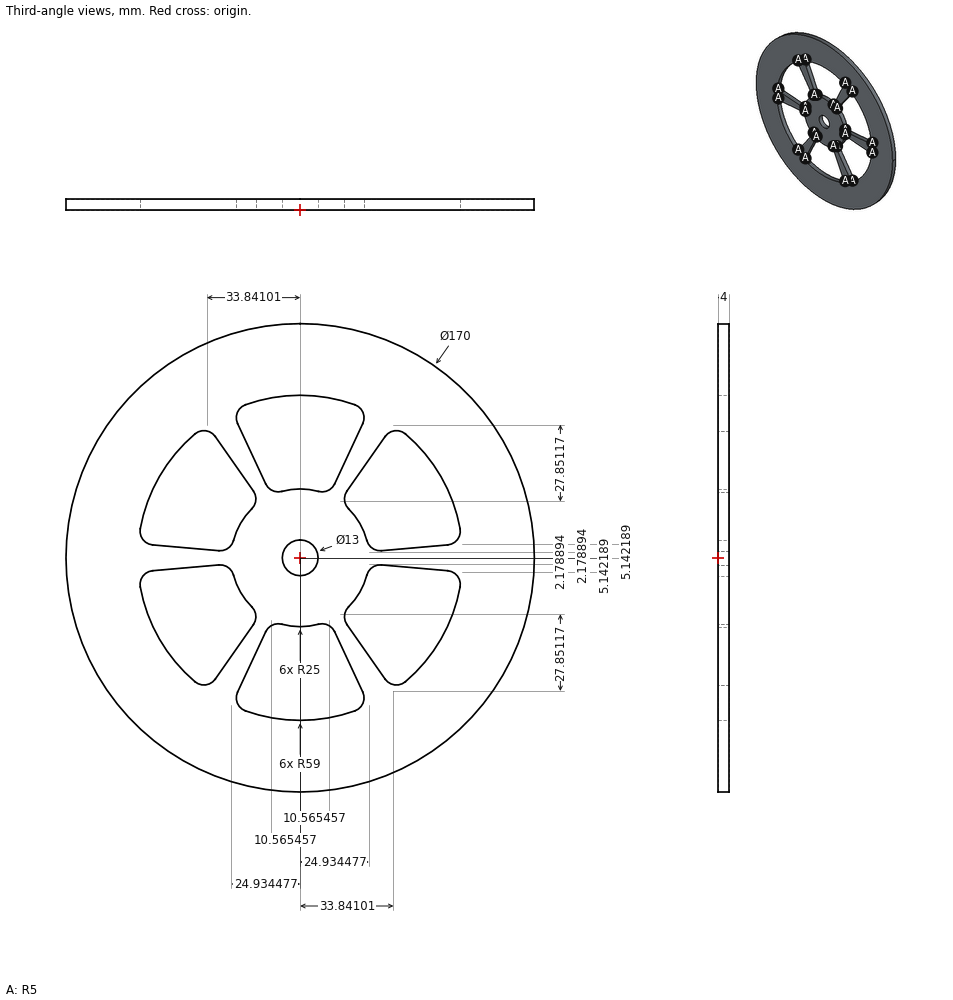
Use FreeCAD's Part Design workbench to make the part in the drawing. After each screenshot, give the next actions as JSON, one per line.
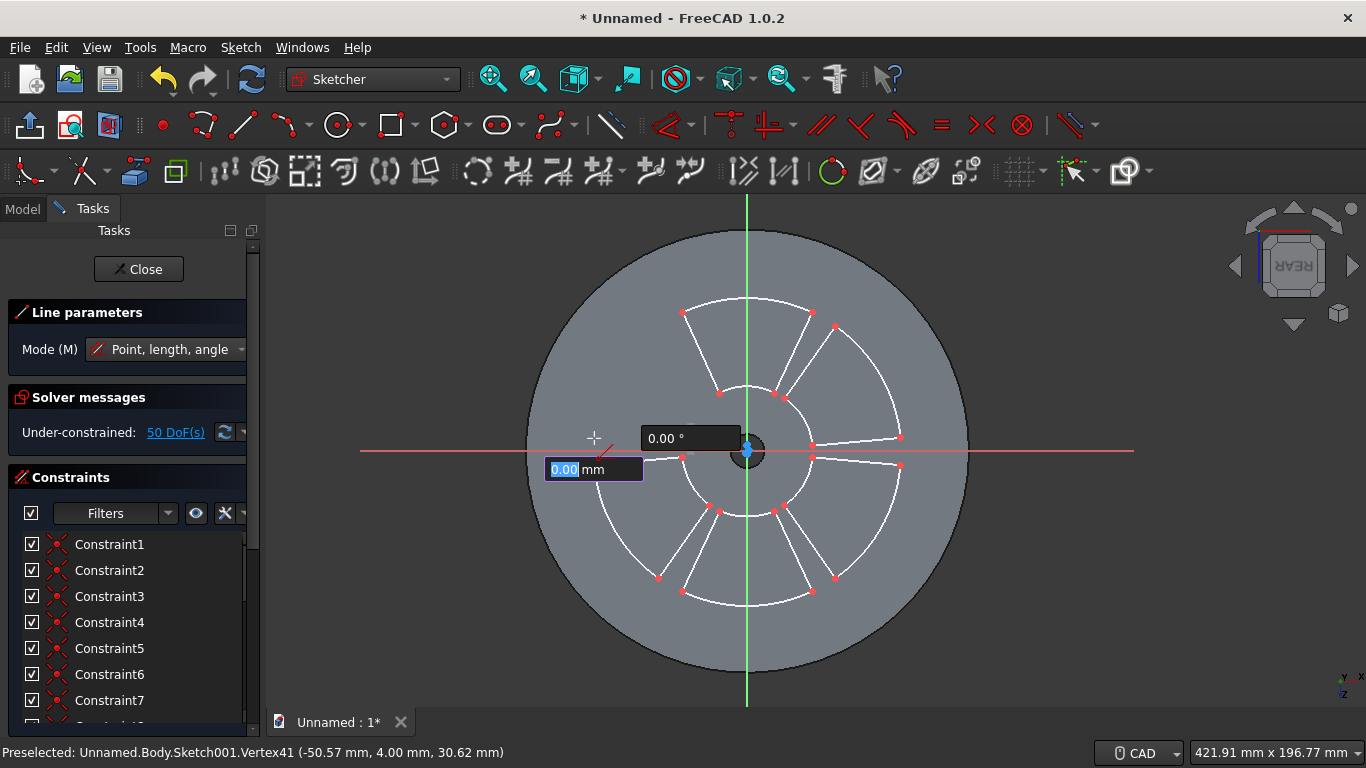
{"action": "scroll", "coordinate": [682, 445], "scroll_direction": "up", "scroll_amount": 6}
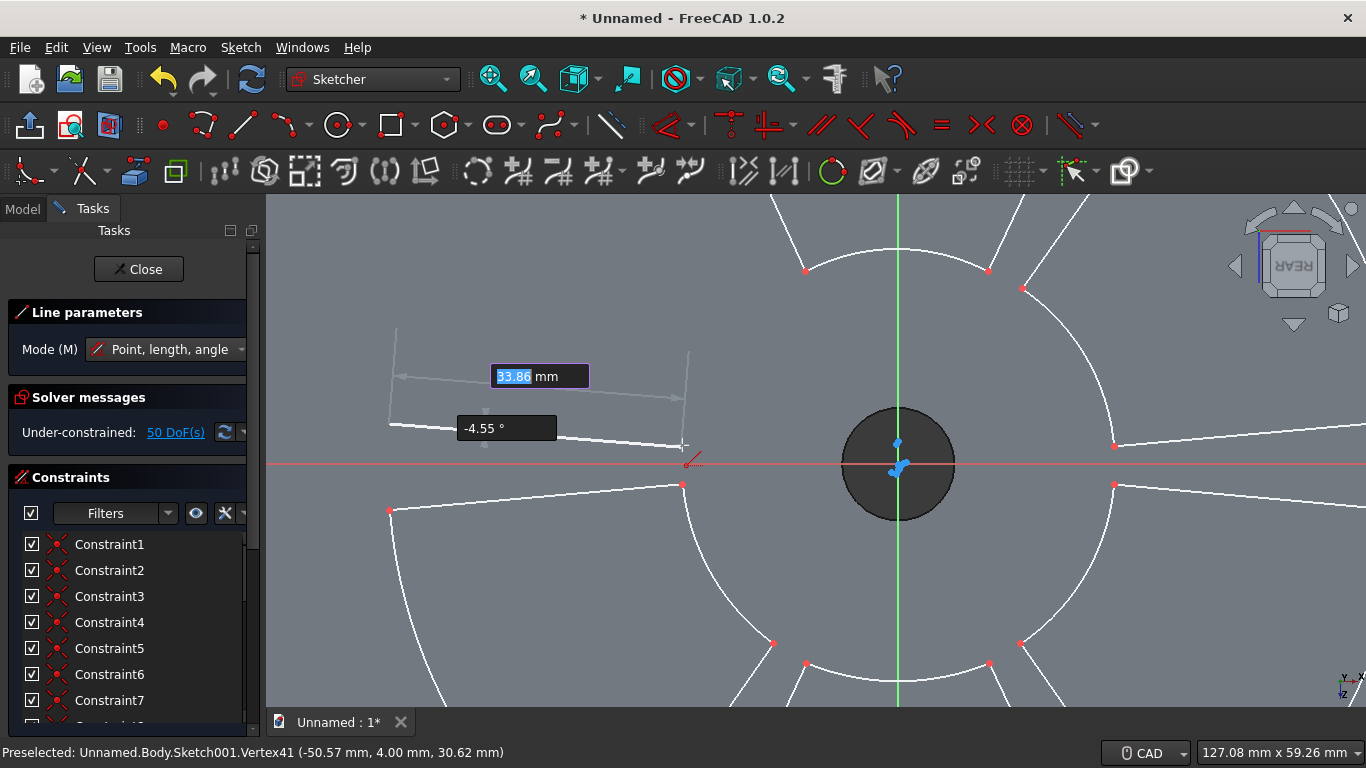
{"action": "left_click", "coordinate": [683, 445]}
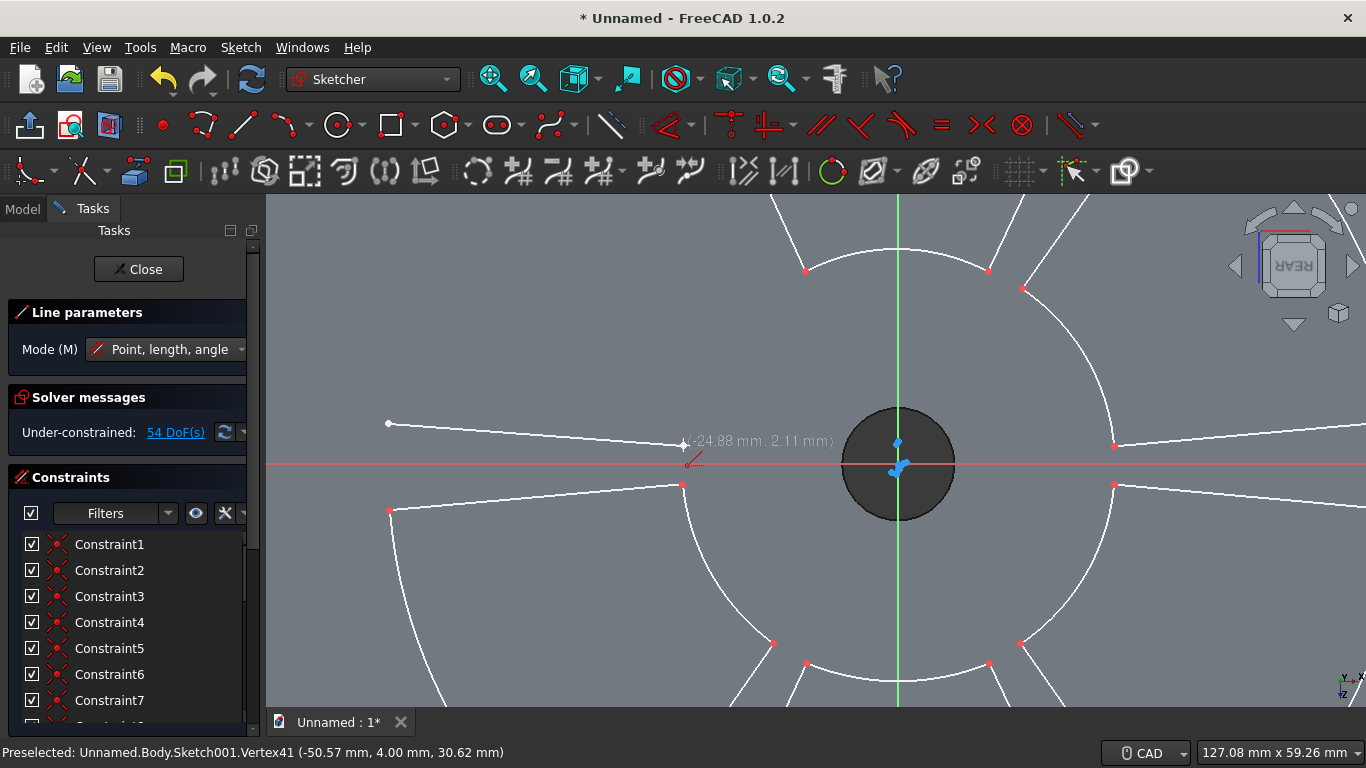
{"action": "left_click", "coordinate": [774, 287]}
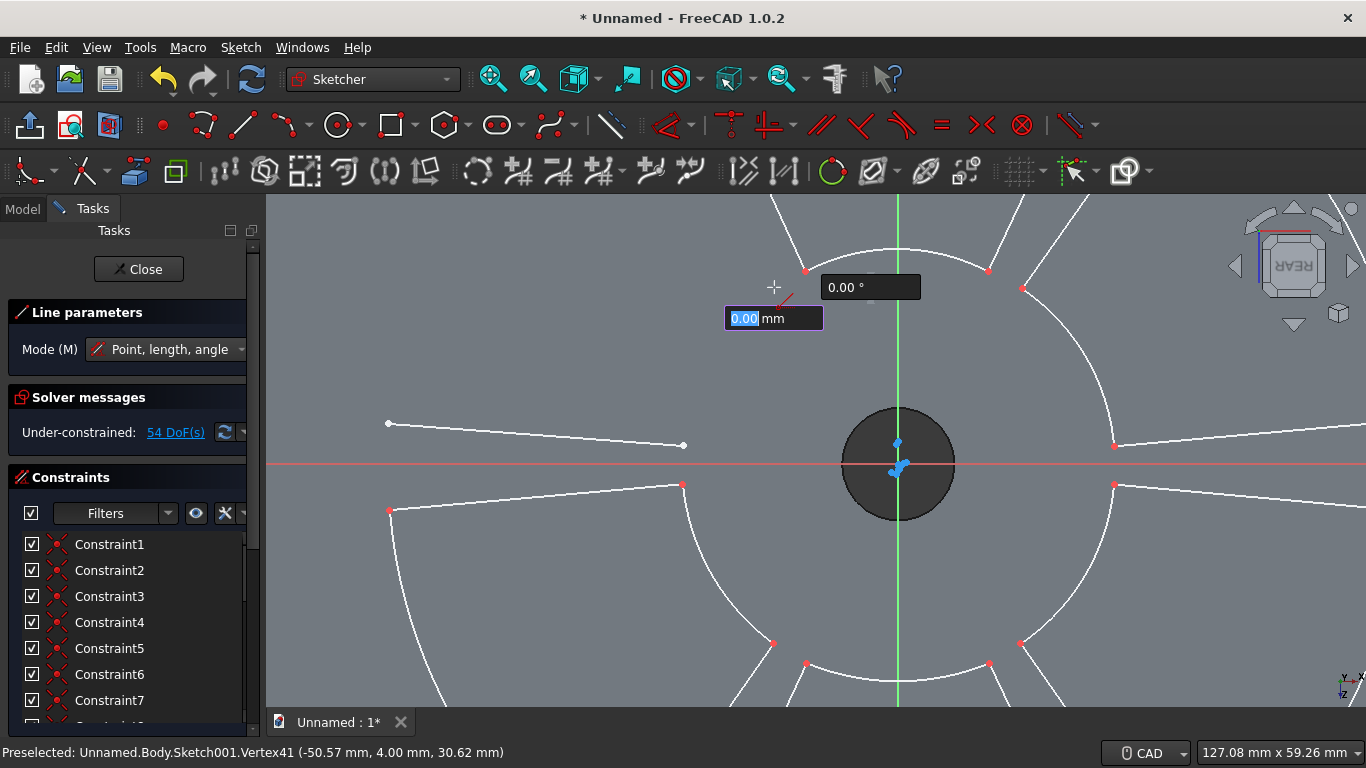
{"action": "scroll", "coordinate": [682, 445], "scroll_direction": "down", "scroll_amount": 6}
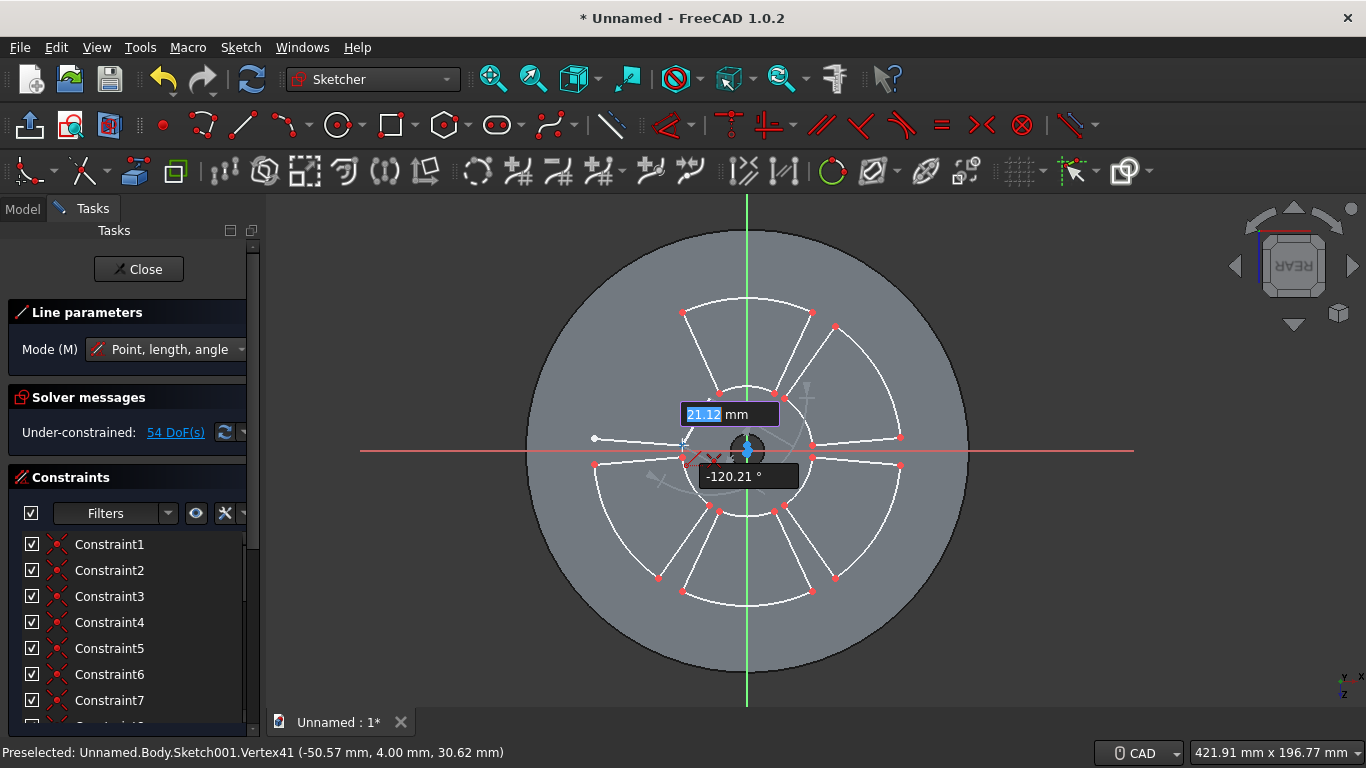
{"action": "left_click", "coordinate": [659, 325]}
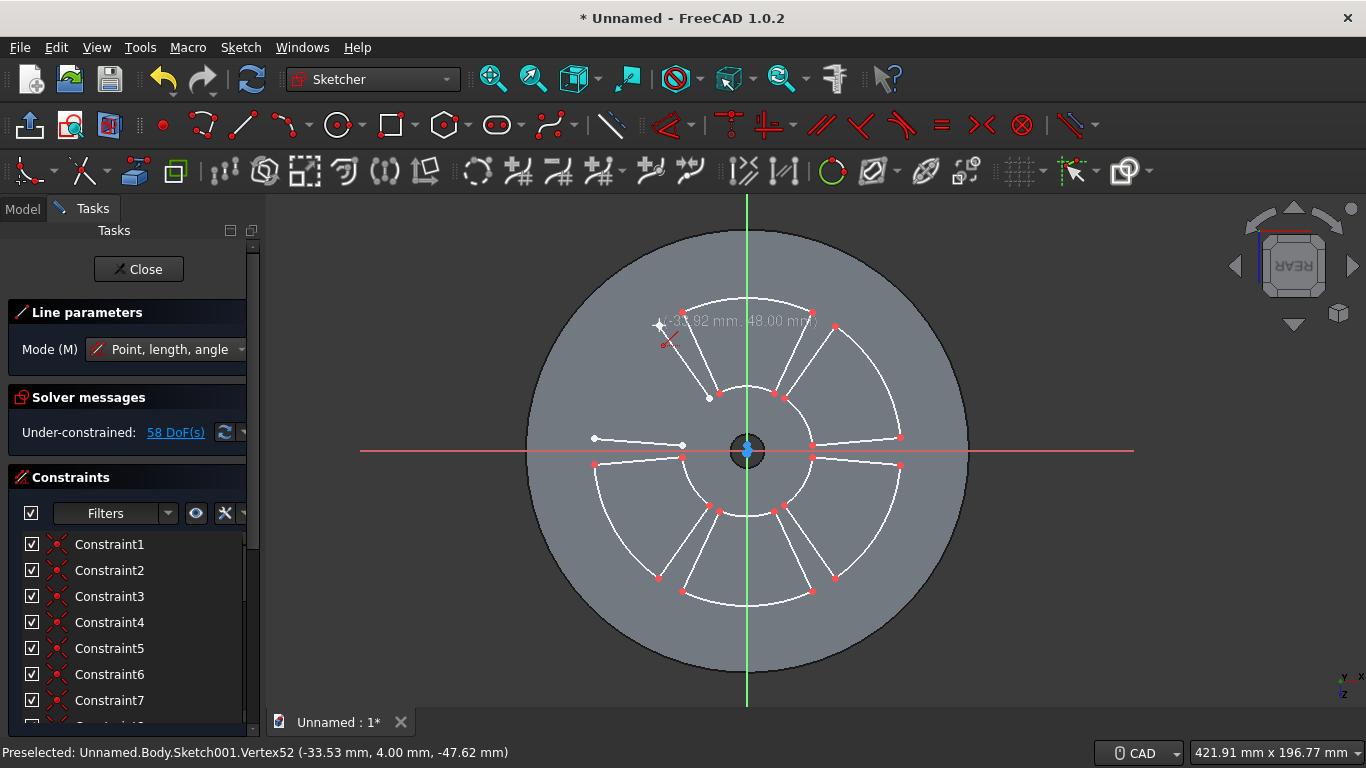
{"action": "left_click", "coordinate": [284, 126]}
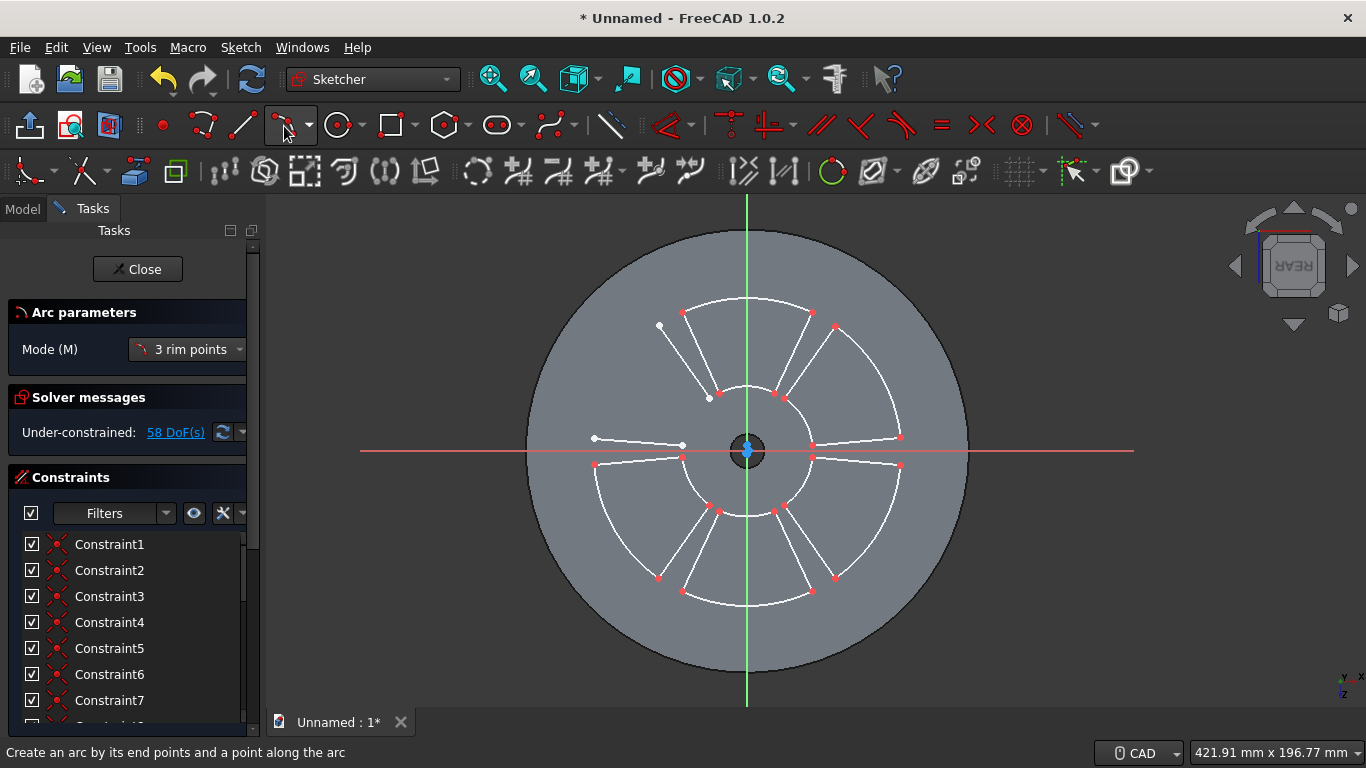
{"action": "scroll", "coordinate": [682, 445], "scroll_direction": "up", "scroll_amount": 6}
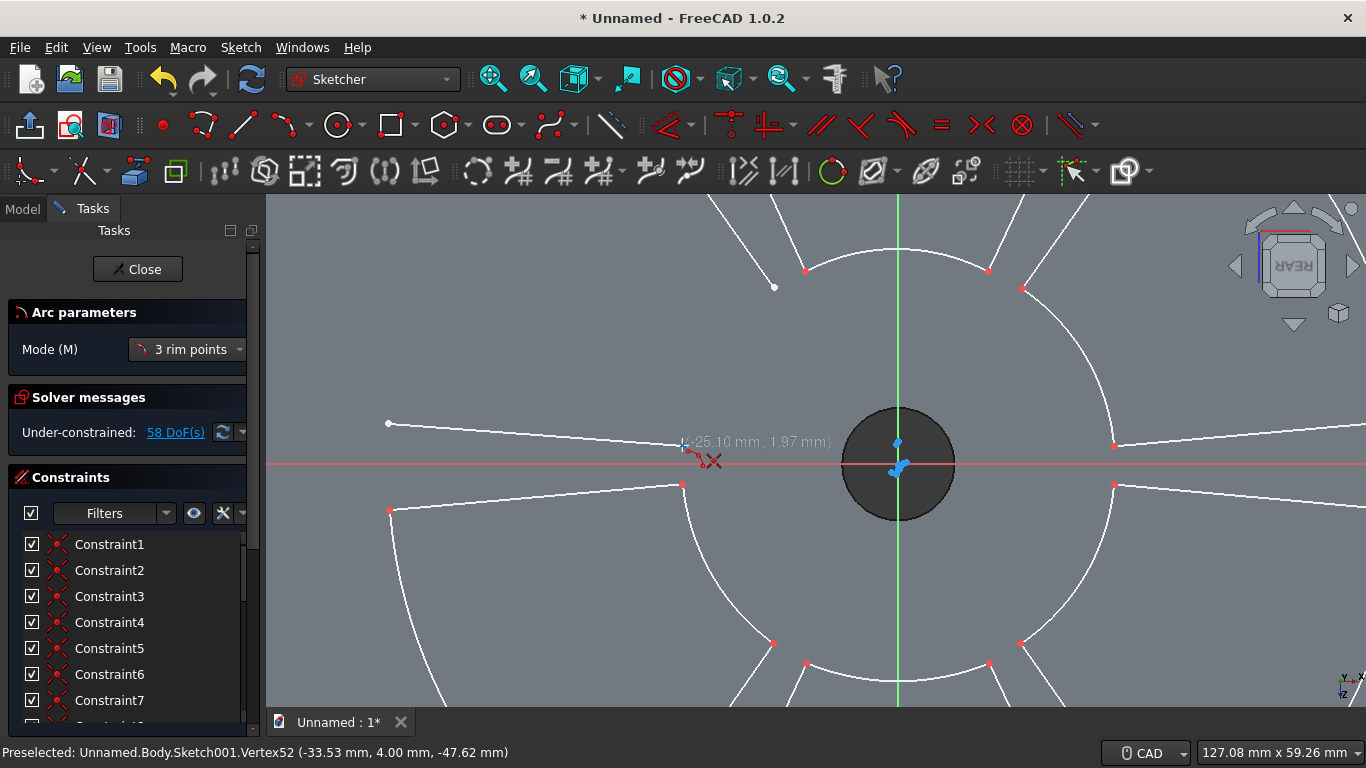
{"action": "left_click", "coordinate": [683, 446]}
{"action": "left_click", "coordinate": [774, 288]}
{"action": "left_click", "coordinate": [711, 356]}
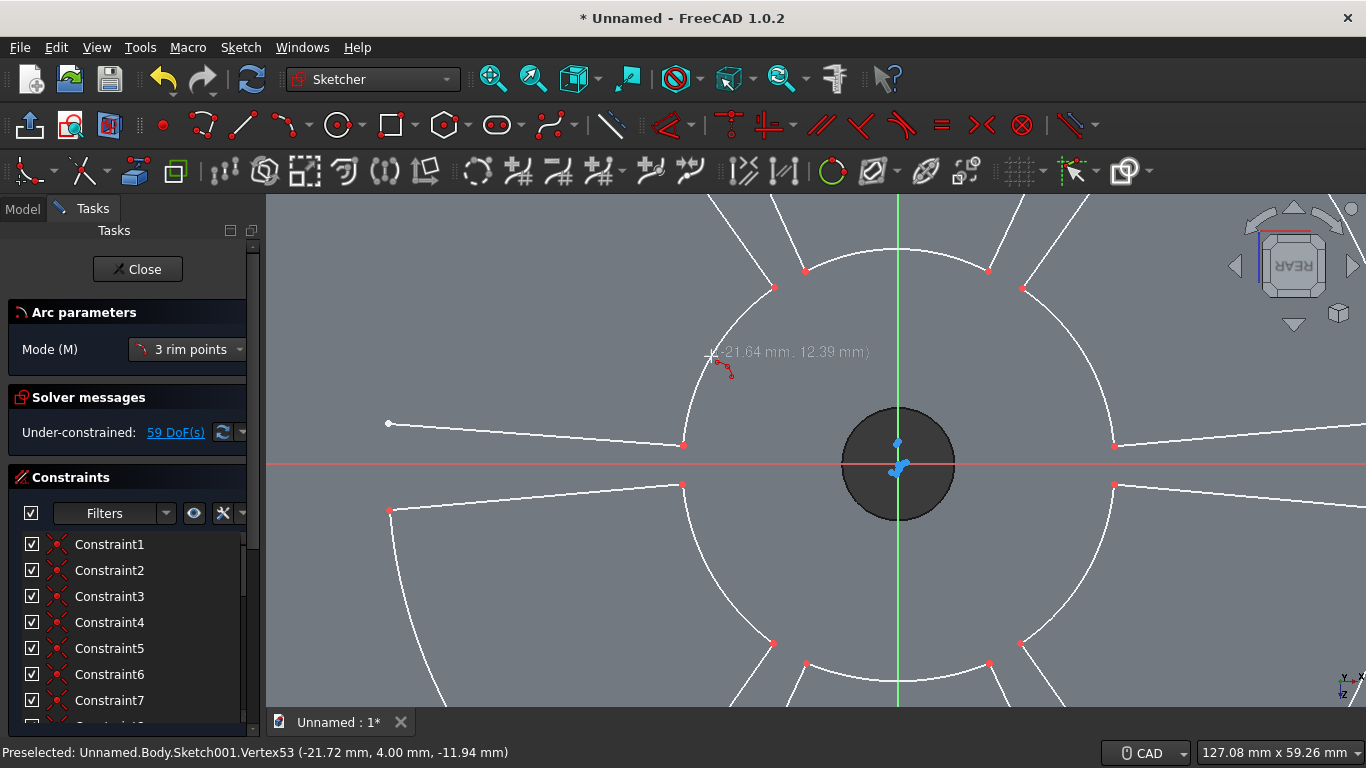
{"action": "scroll", "coordinate": [682, 445], "scroll_direction": "down", "scroll_amount": 6}